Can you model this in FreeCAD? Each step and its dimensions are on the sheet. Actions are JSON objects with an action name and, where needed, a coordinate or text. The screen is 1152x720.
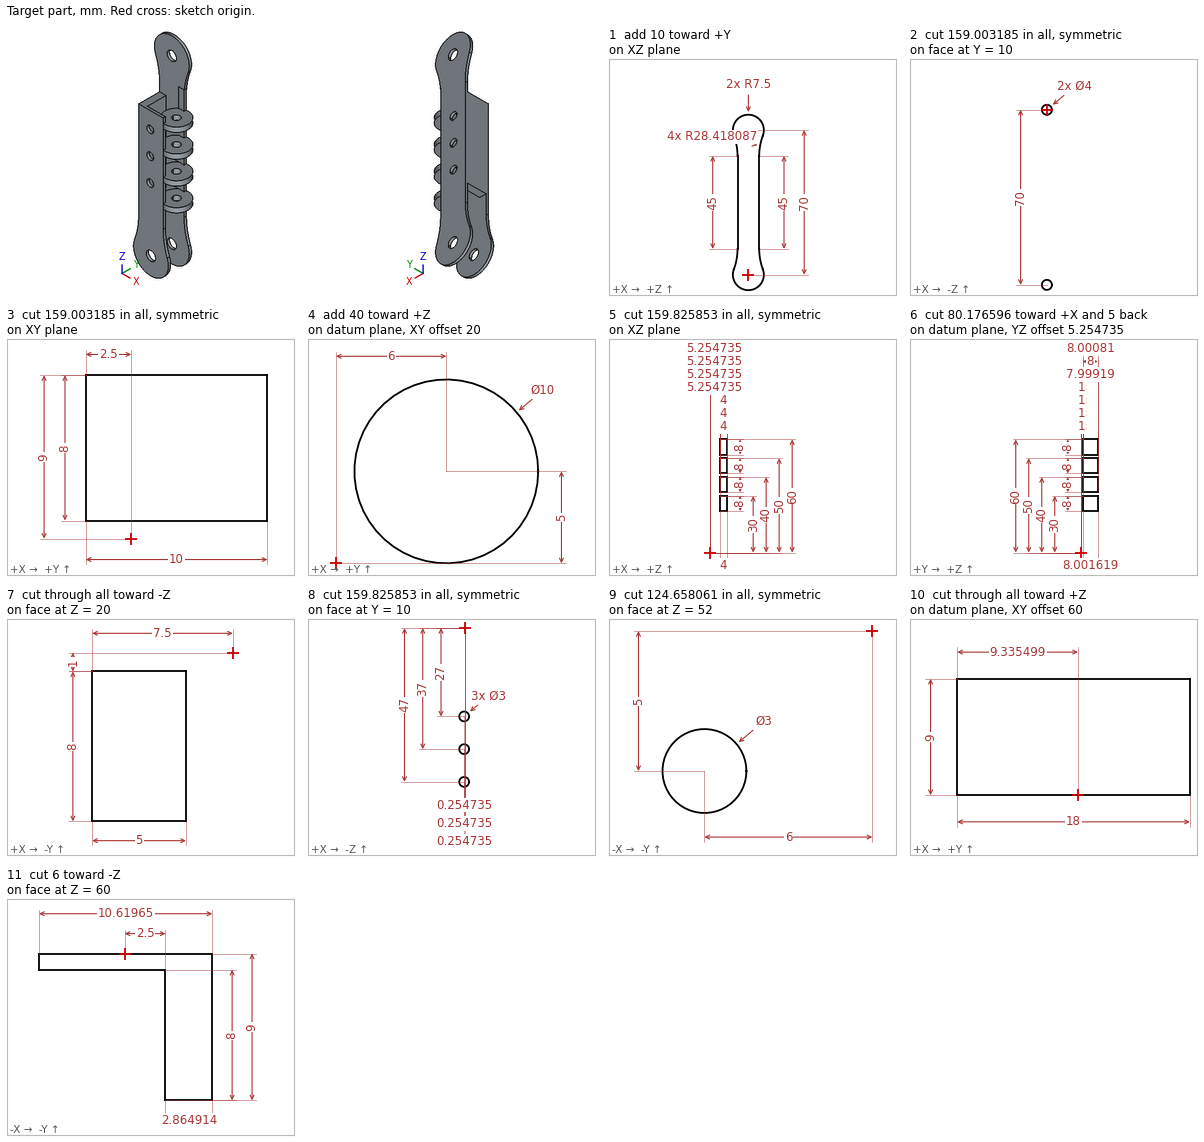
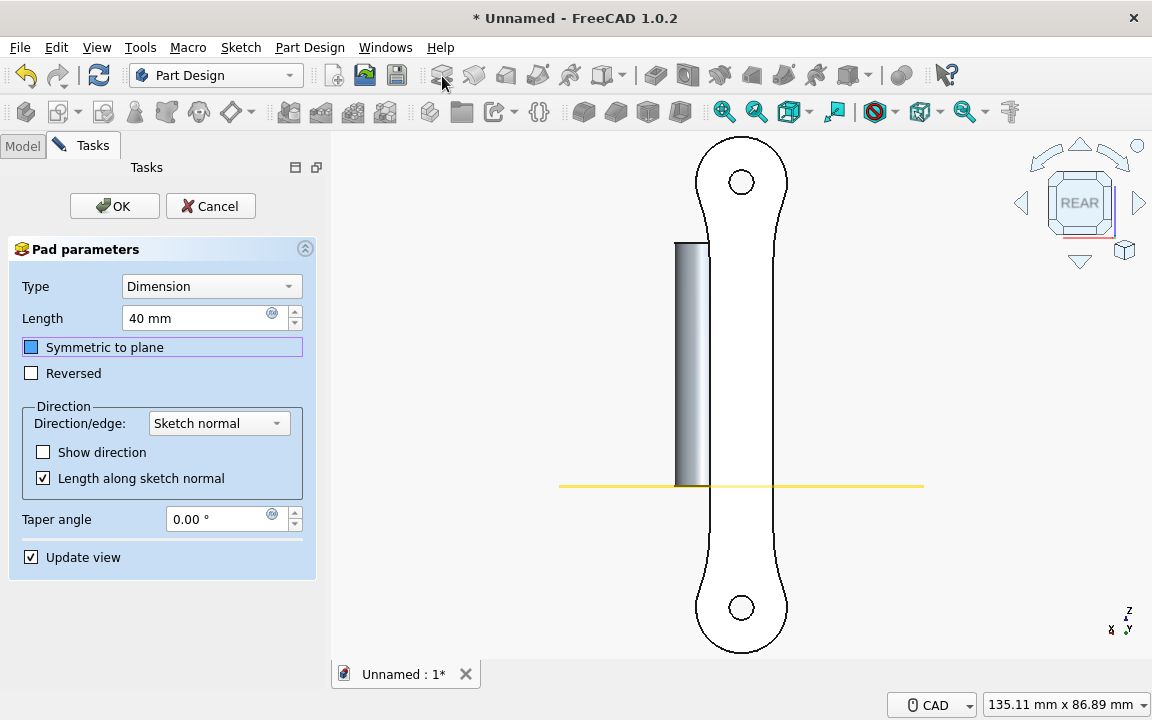
{"action": "left_click", "coordinate": [115, 206]}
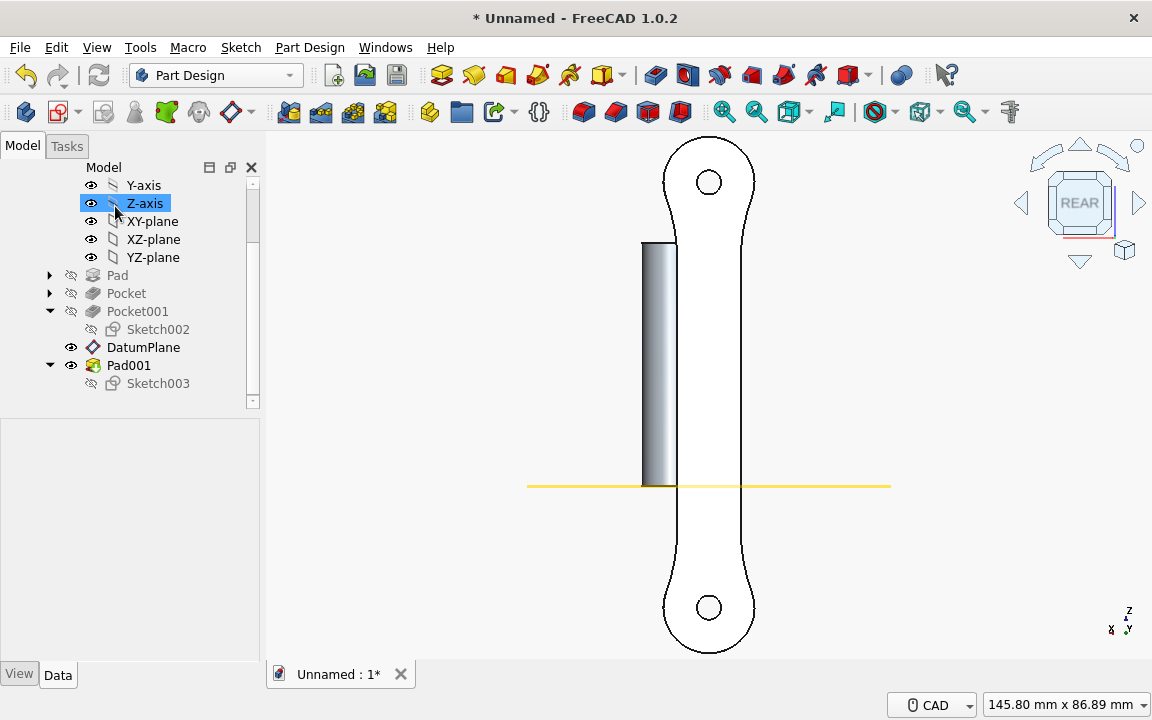
{"action": "left_click", "coordinate": [116, 347]}
{"action": "key", "text": "space"}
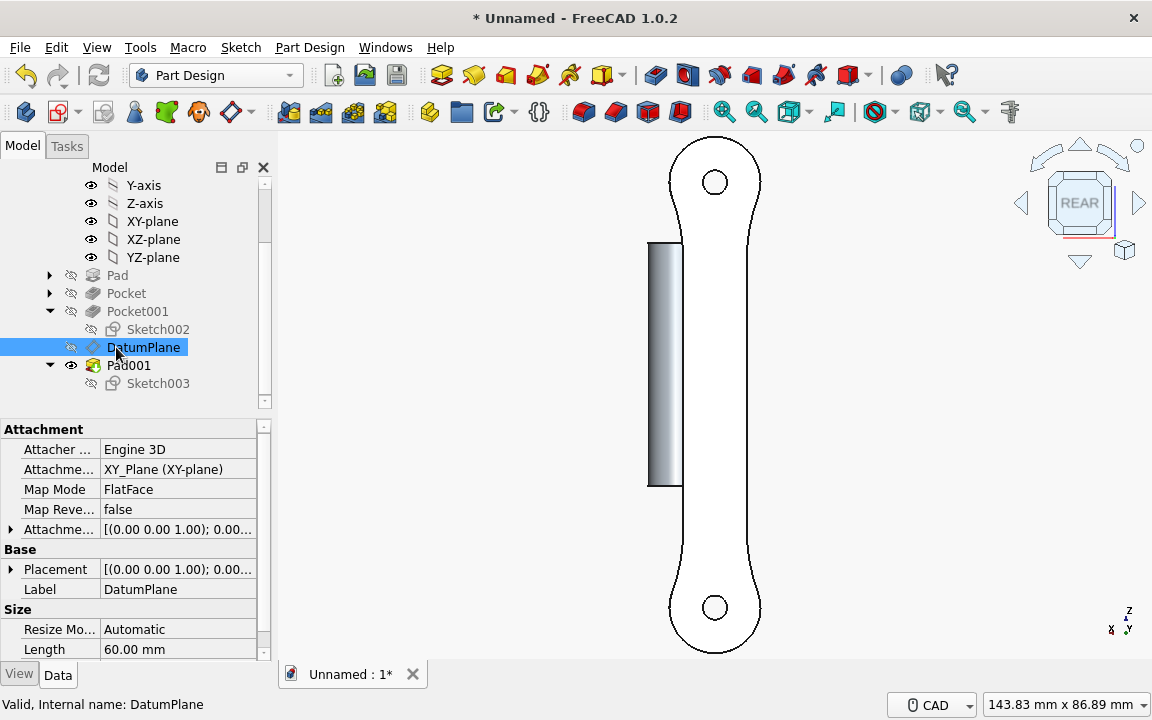
{"action": "left_click", "coordinate": [318, 619]}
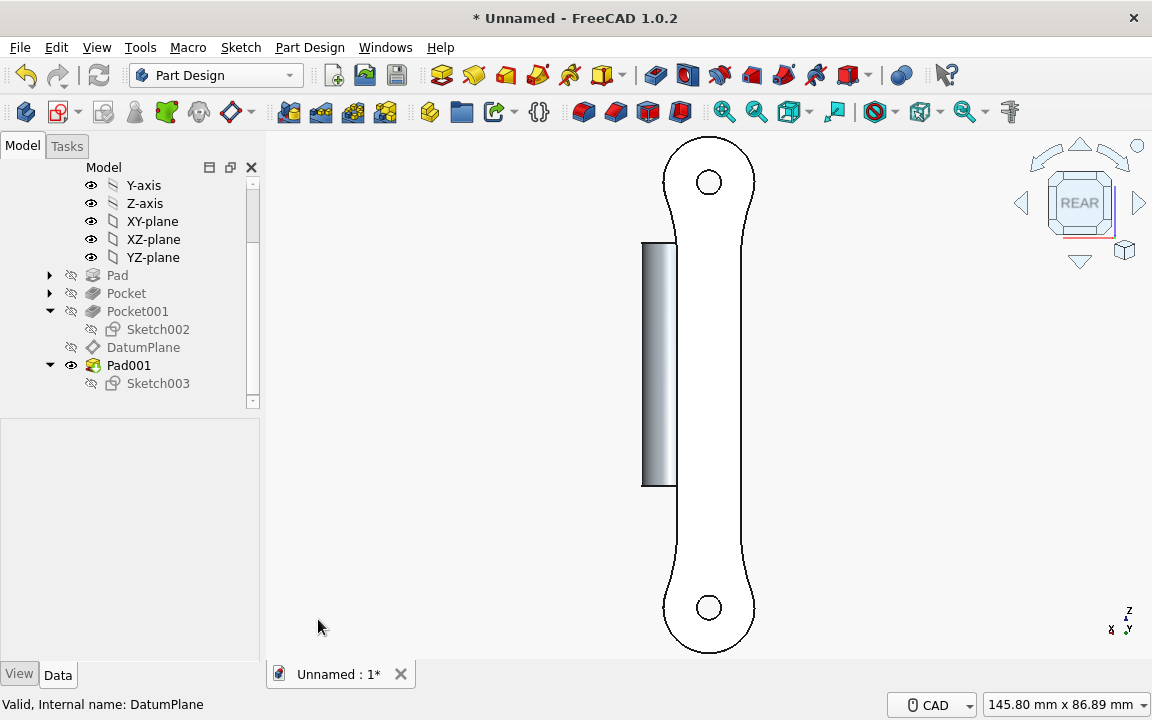
{"action": "left_click", "coordinate": [58, 112]}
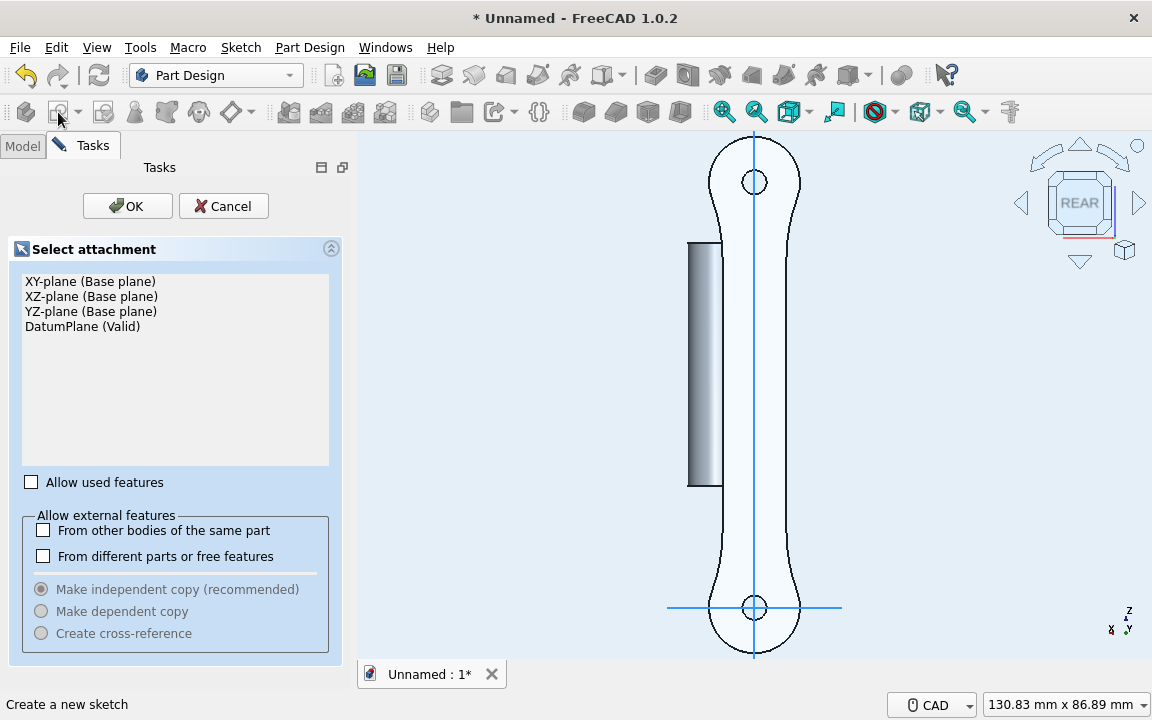
{"action": "left_click", "coordinate": [82, 296]}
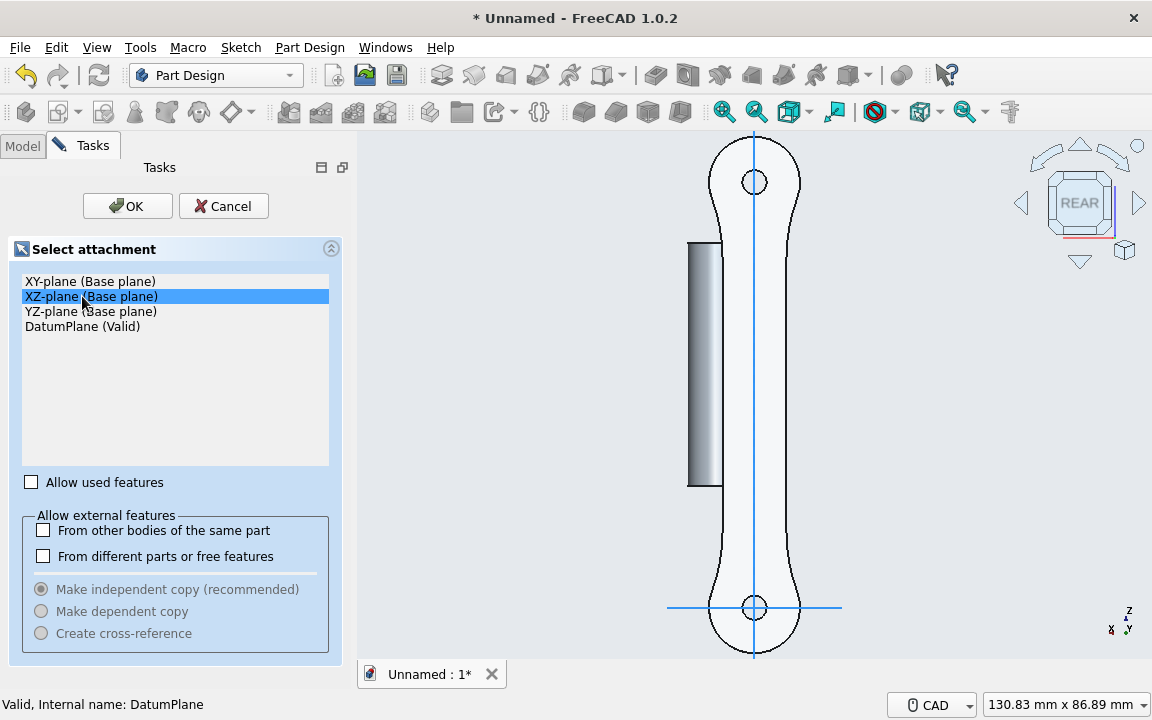
{"action": "left_click", "coordinate": [128, 206]}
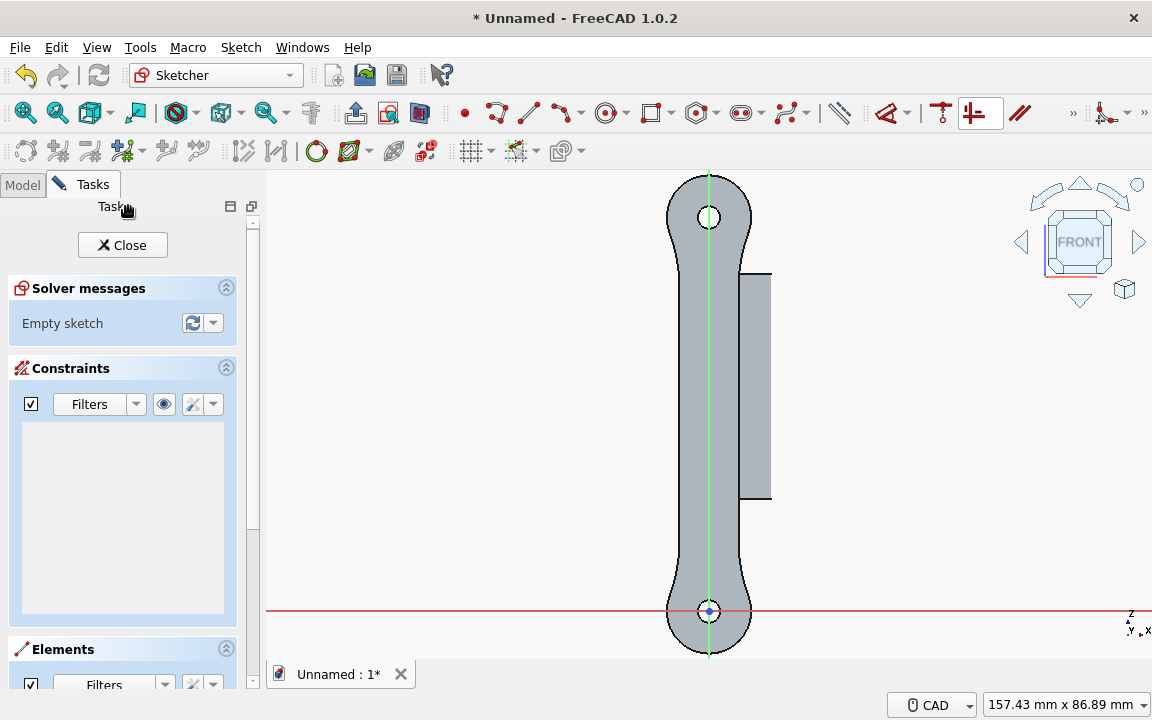
{"action": "scroll", "coordinate": [294, 287], "scroll_direction": "down", "scroll_amount": 1}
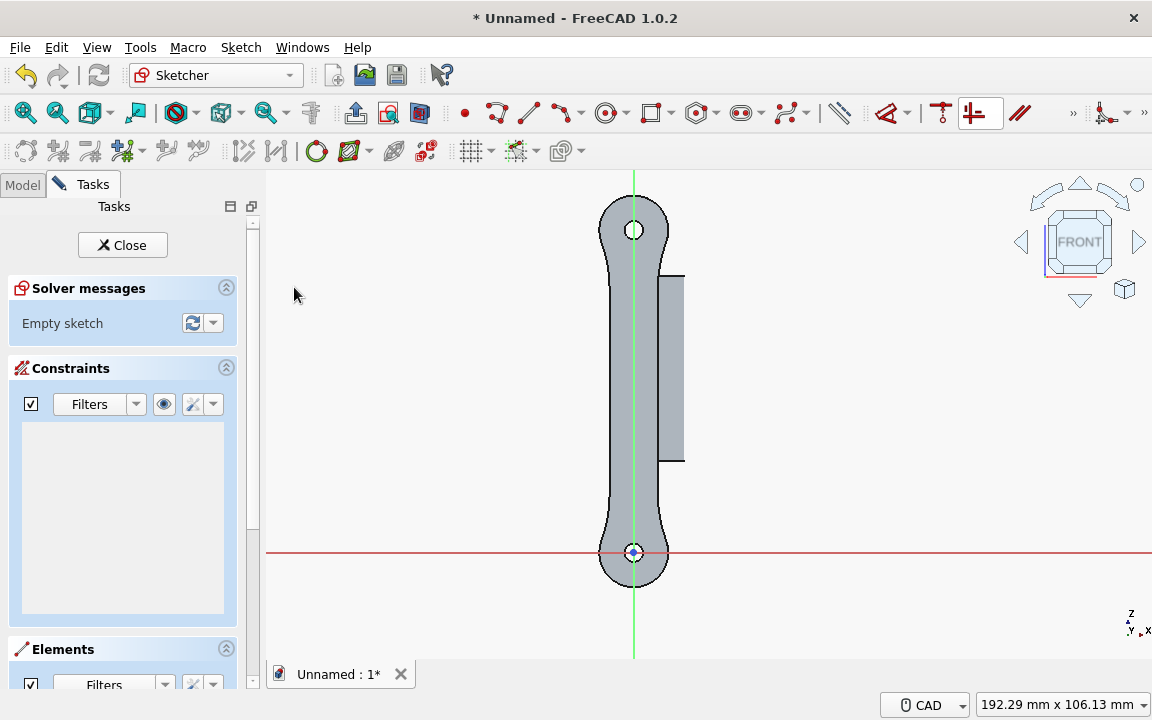
{"action": "left_click", "coordinate": [652, 114]}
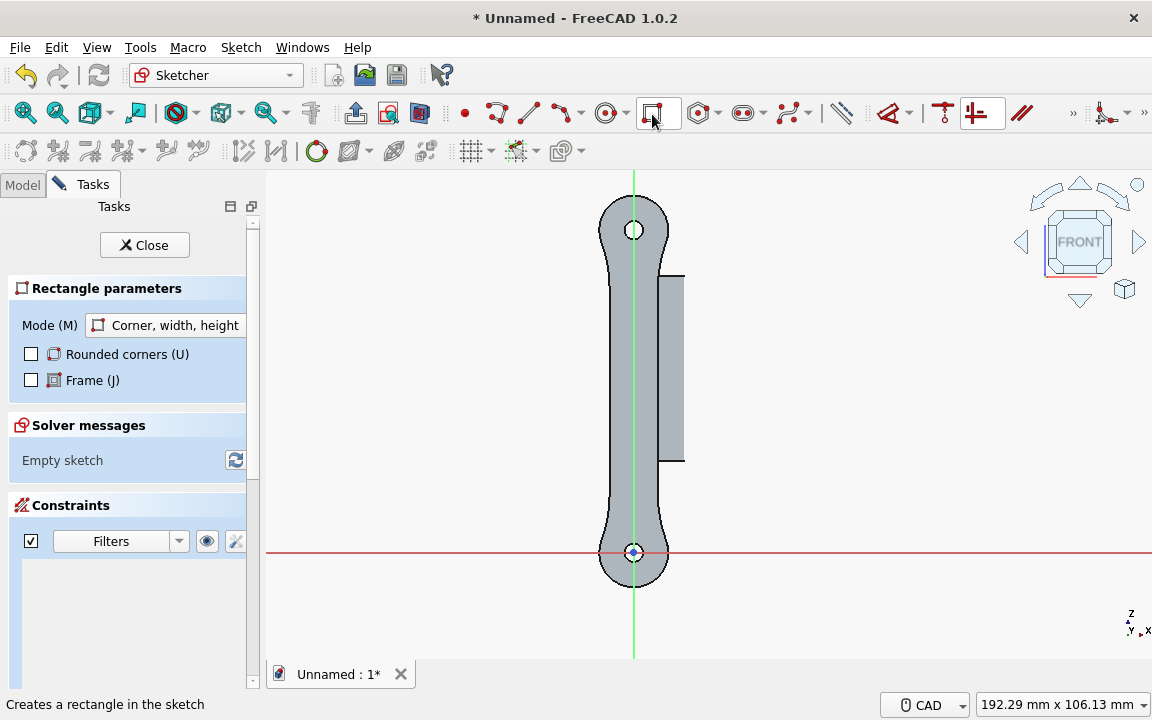
{"action": "left_click", "coordinate": [658, 414]}
{"action": "left_click", "coordinate": [676, 451]}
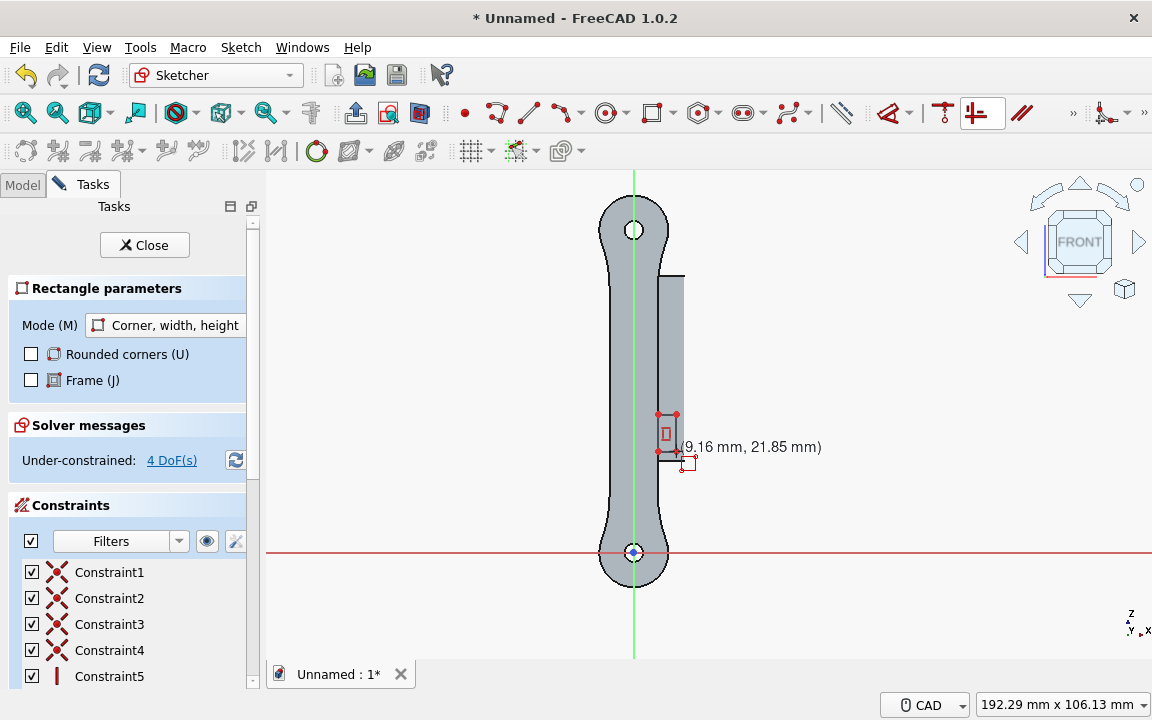
{"action": "left_click", "coordinate": [658, 368]}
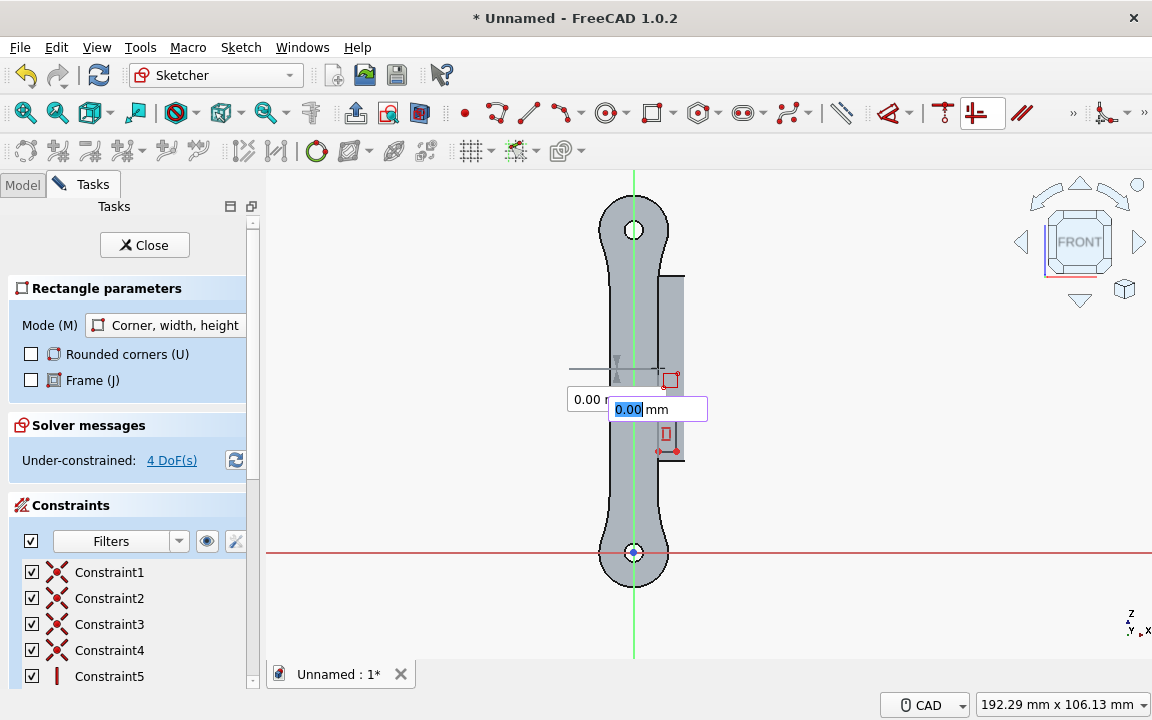
{"action": "scroll", "coordinate": [676, 405], "scroll_direction": "up", "scroll_amount": 3}